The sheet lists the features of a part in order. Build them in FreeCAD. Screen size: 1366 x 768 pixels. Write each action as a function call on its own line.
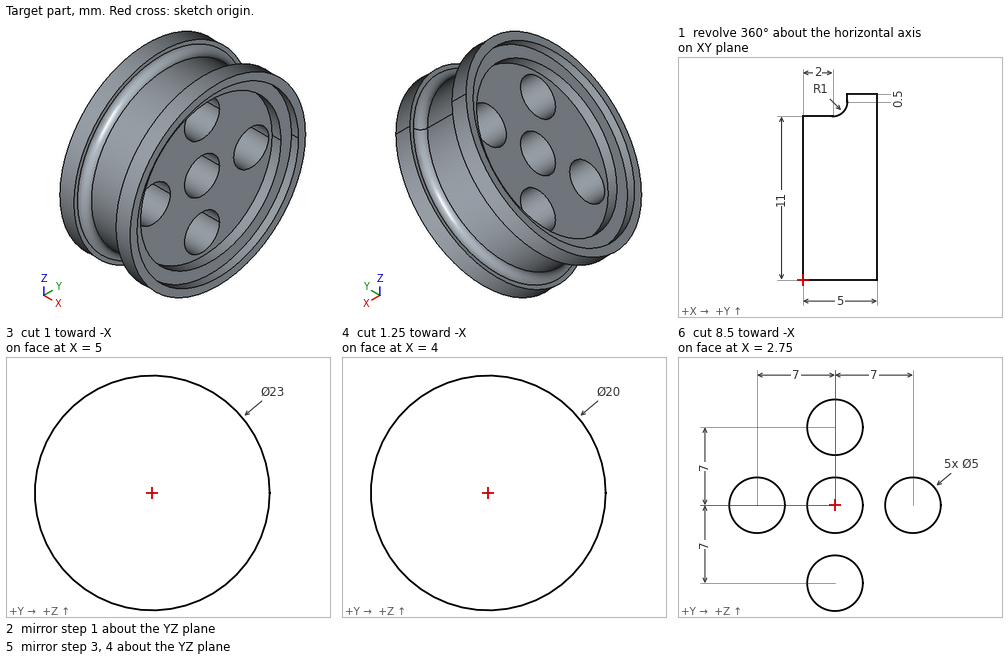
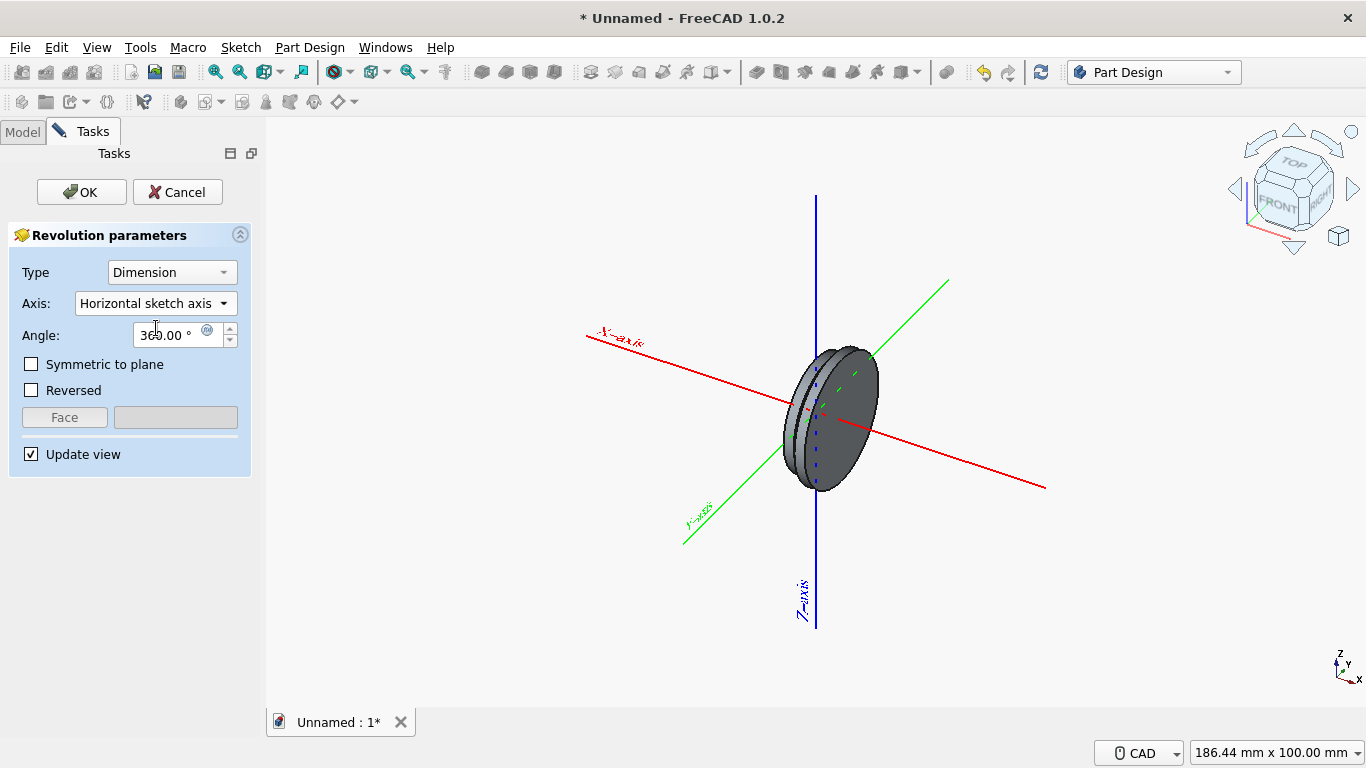
click(82, 192)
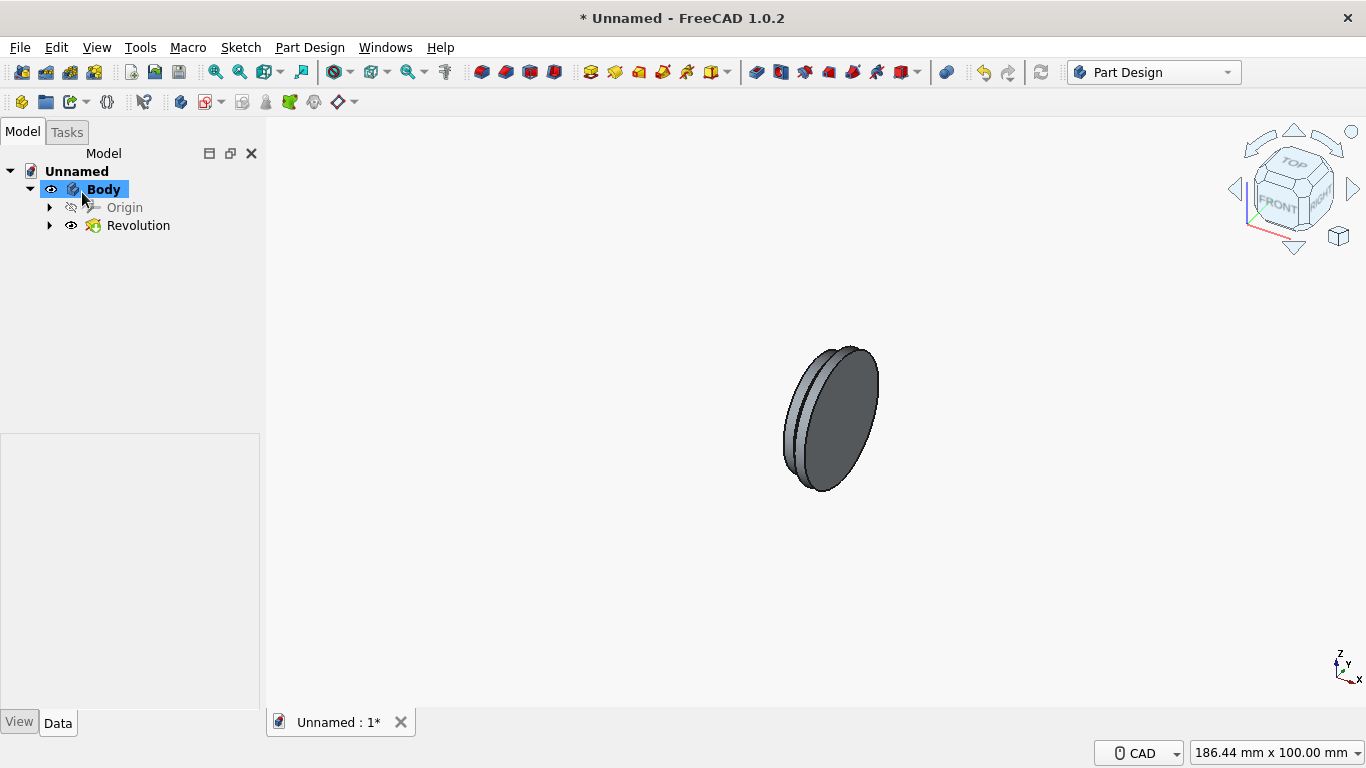
key(v)
key(f)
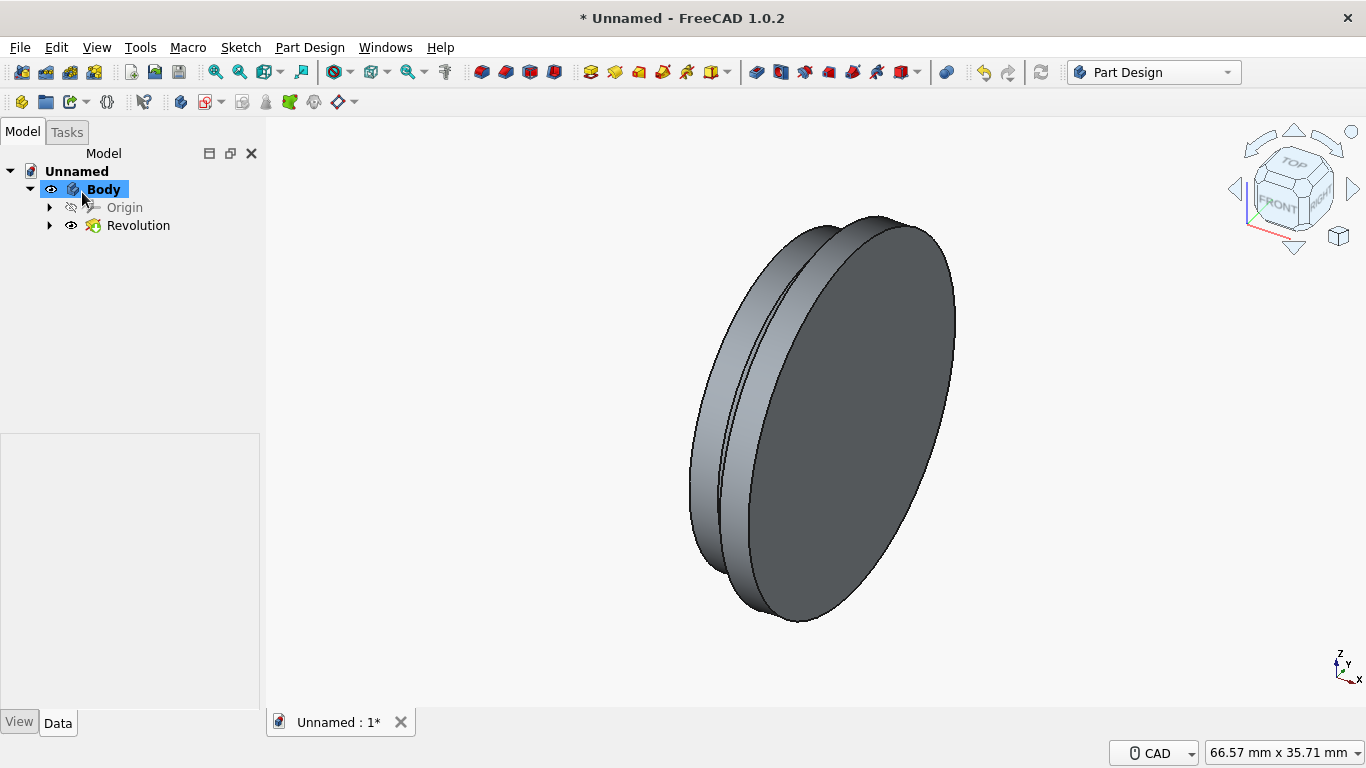
click(116, 225)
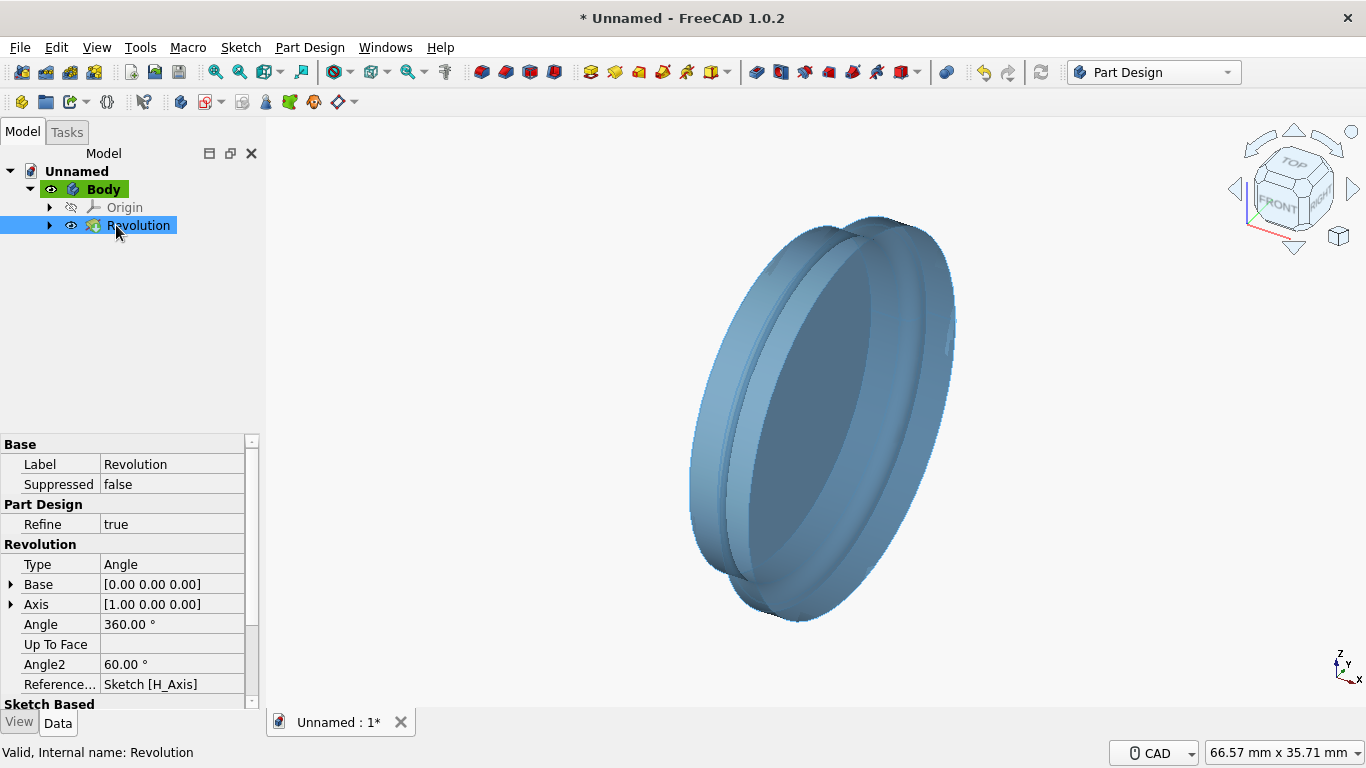
click(22, 72)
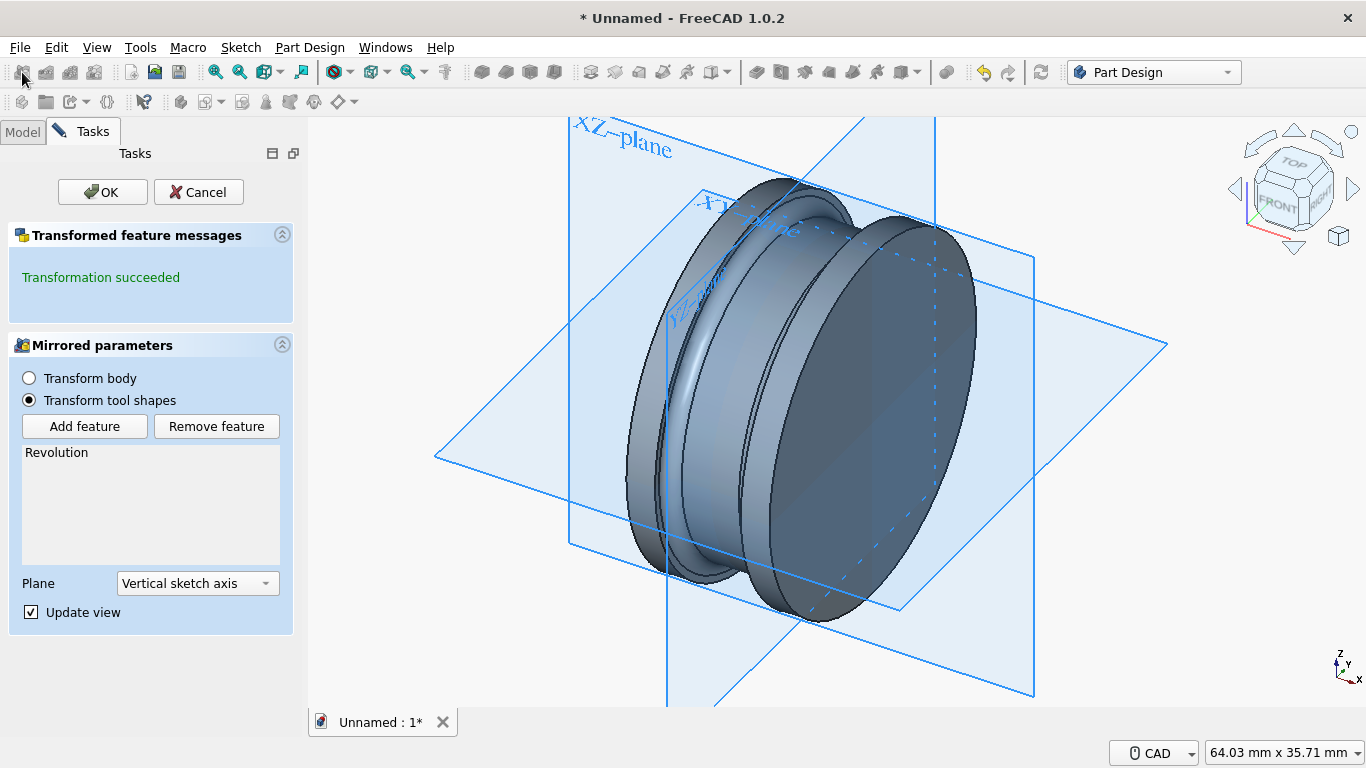
click(198, 584)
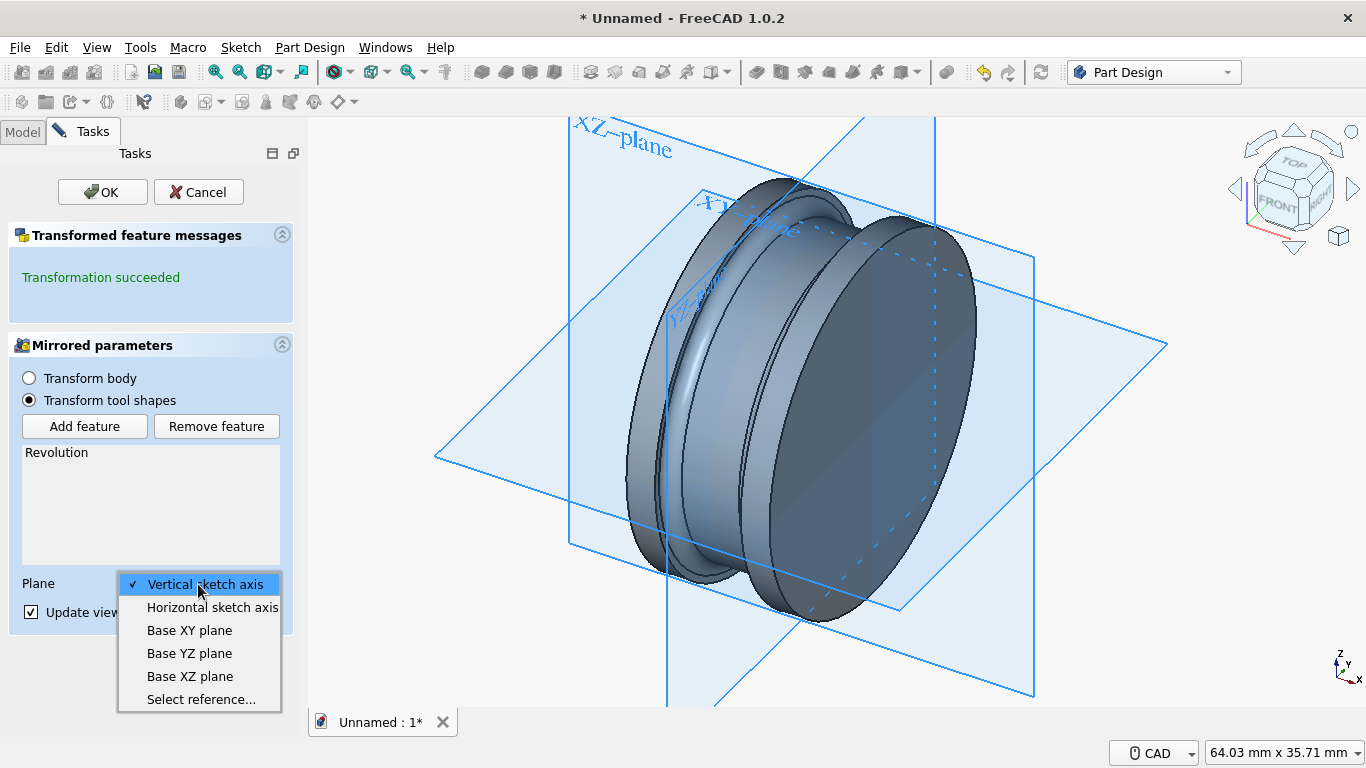
click(198, 654)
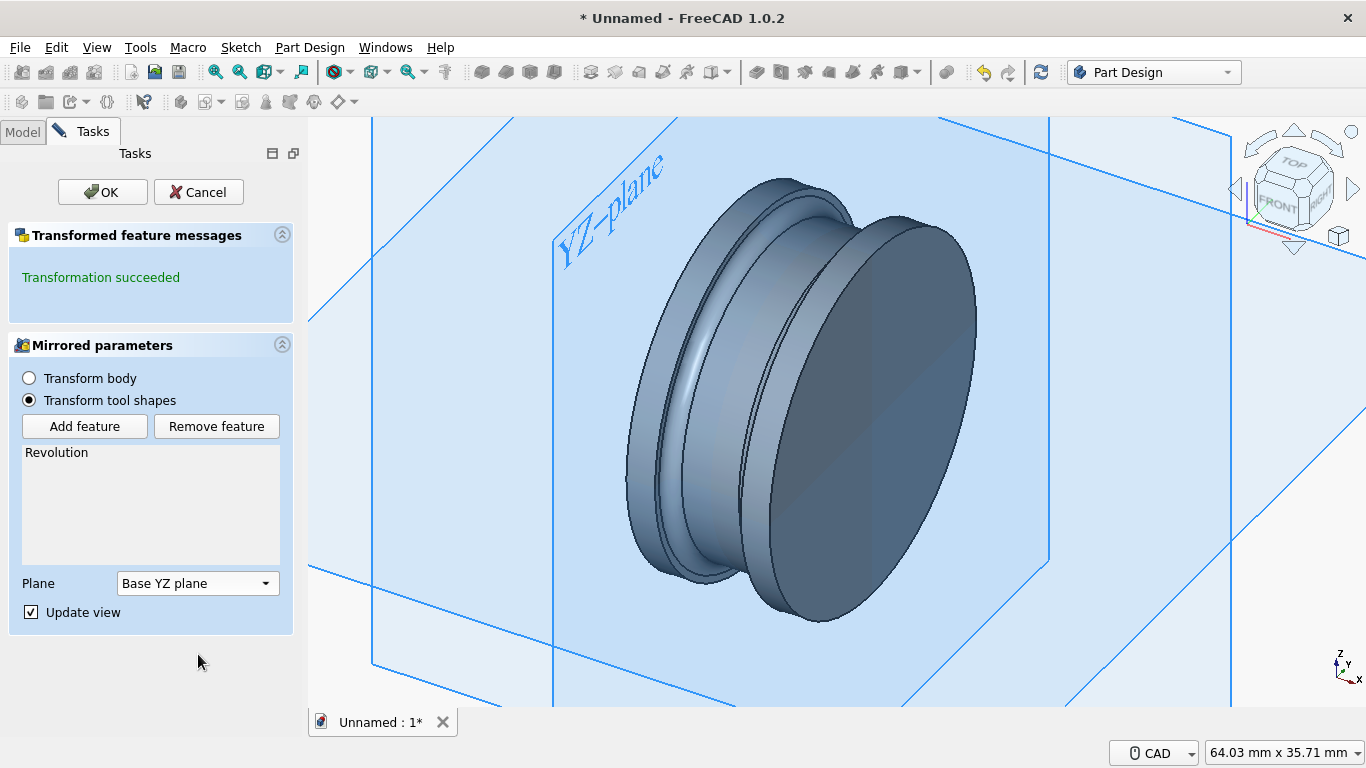
click(103, 192)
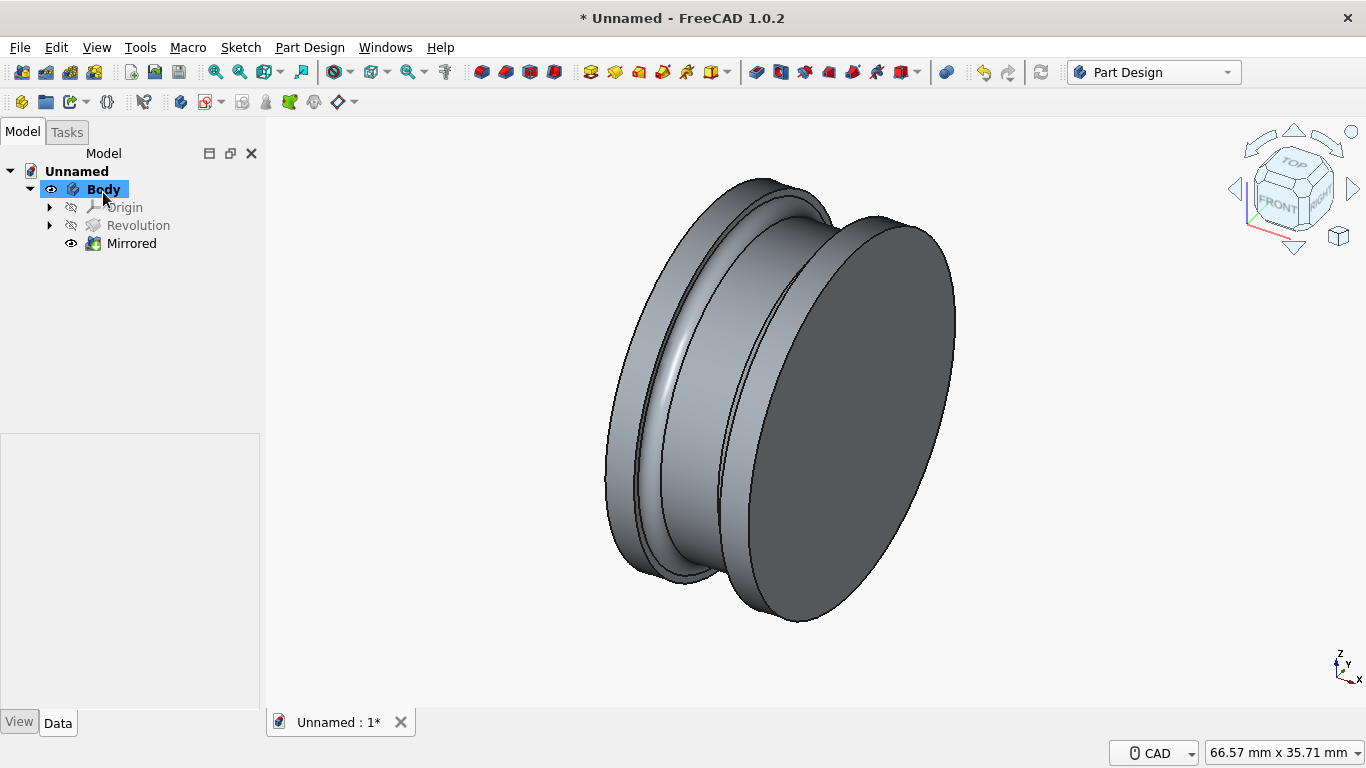
key(v)
key(f)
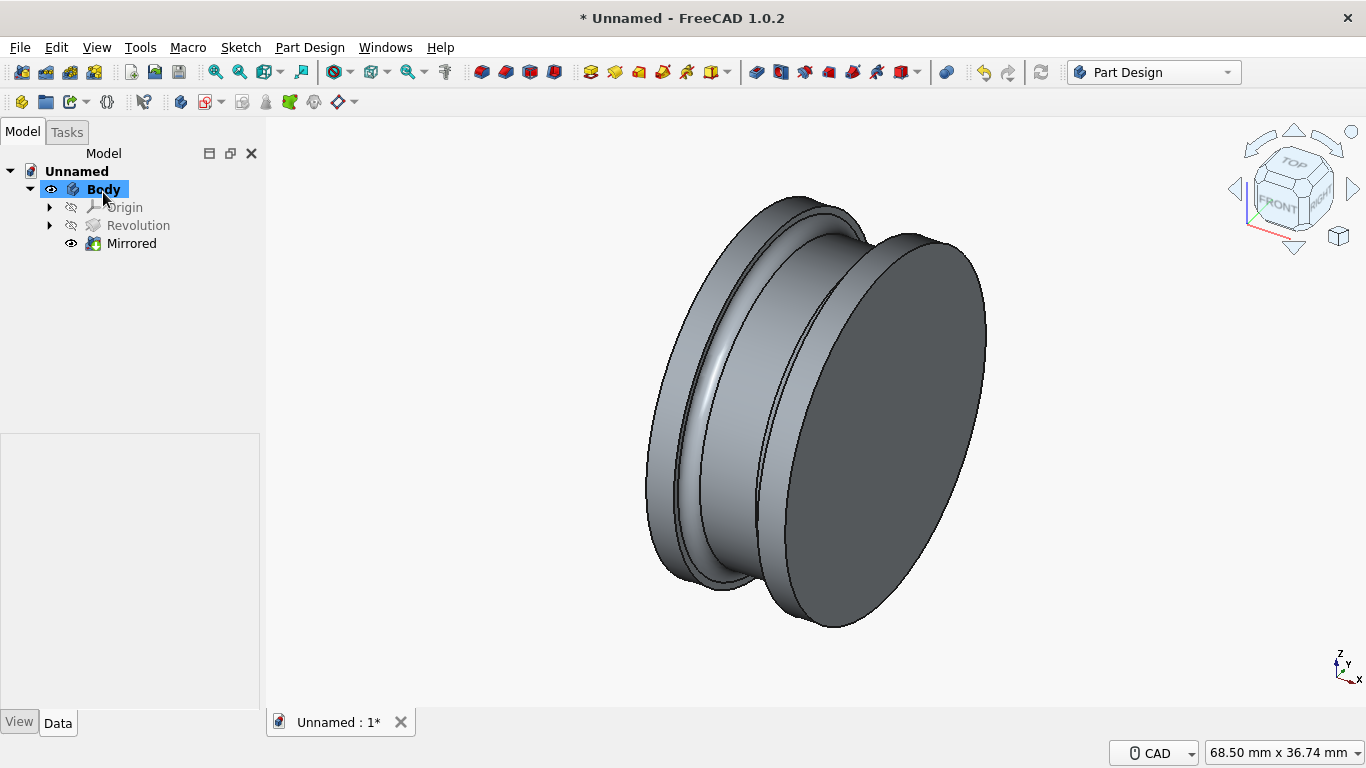
click(886, 434)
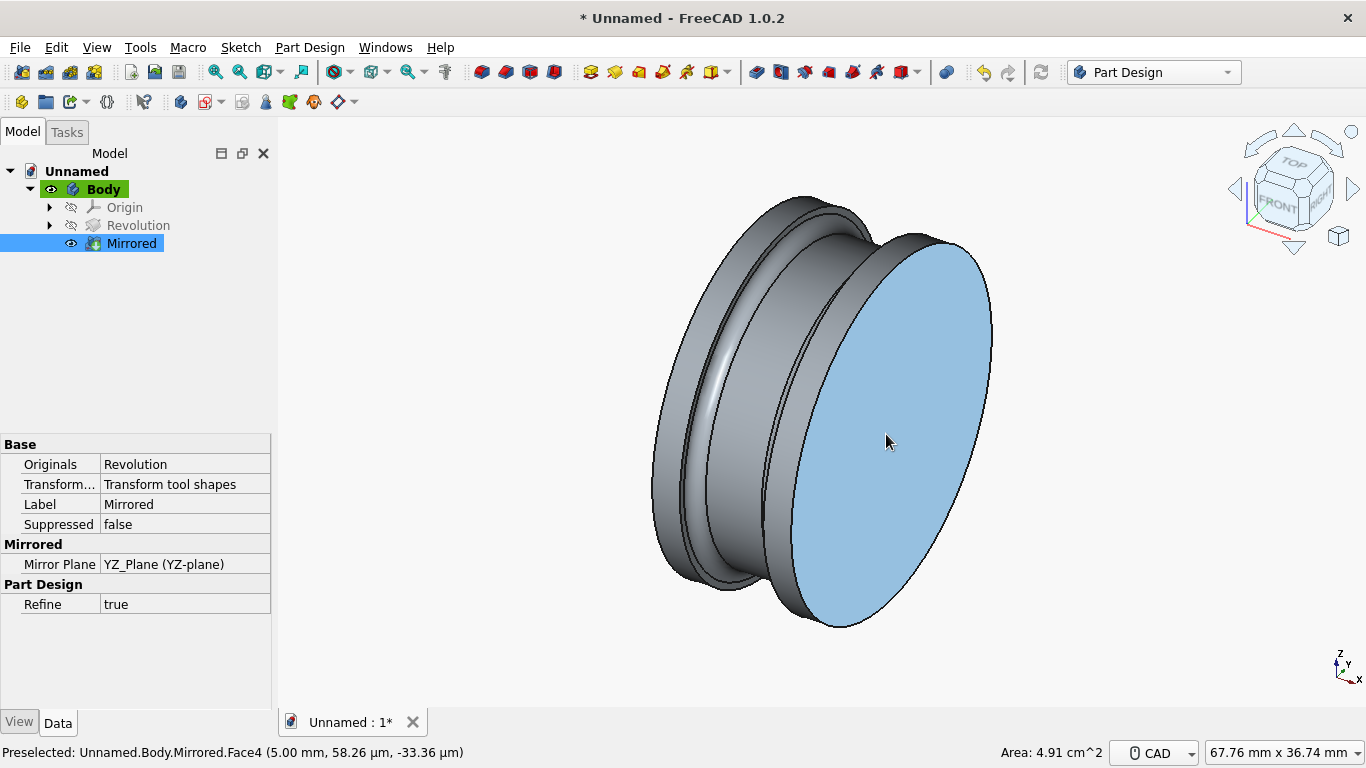
click(206, 102)